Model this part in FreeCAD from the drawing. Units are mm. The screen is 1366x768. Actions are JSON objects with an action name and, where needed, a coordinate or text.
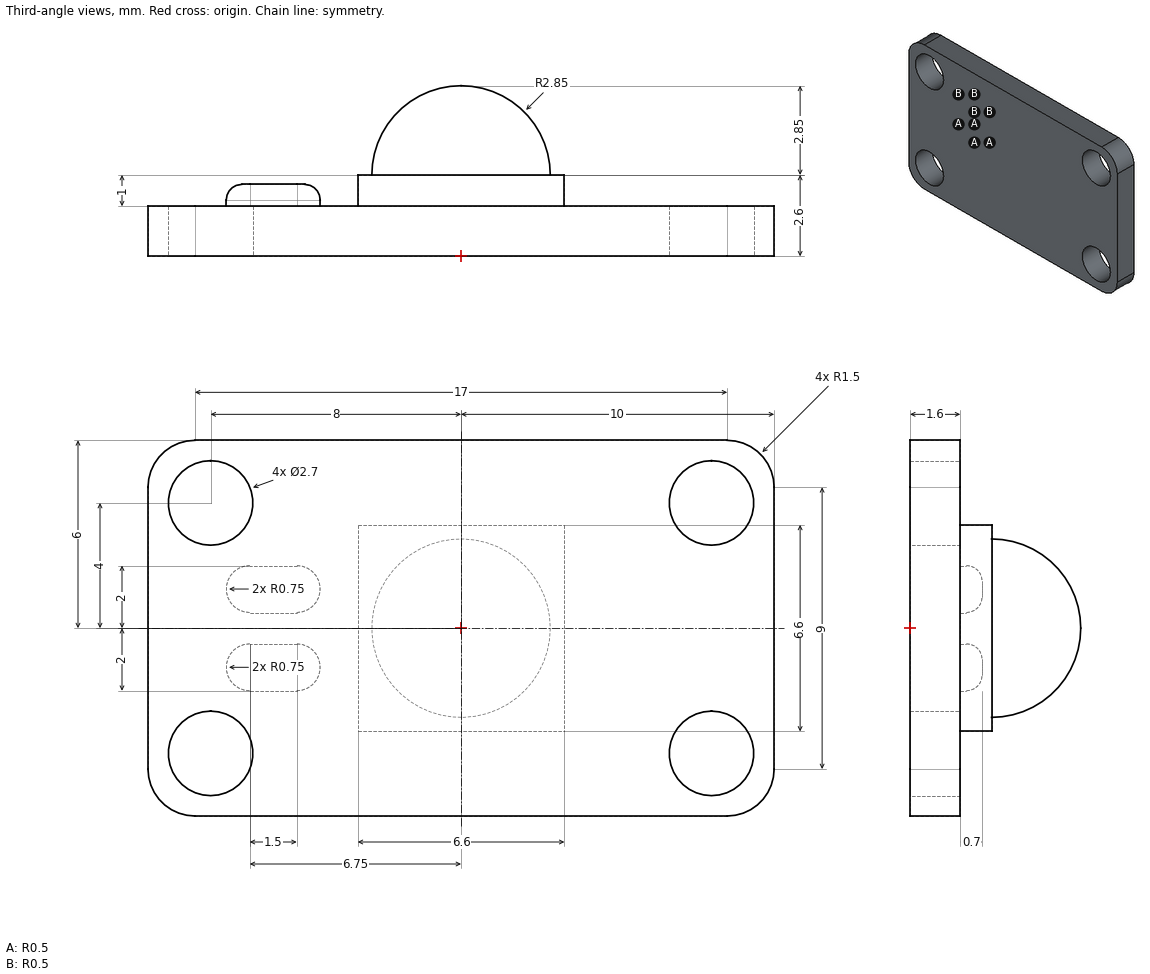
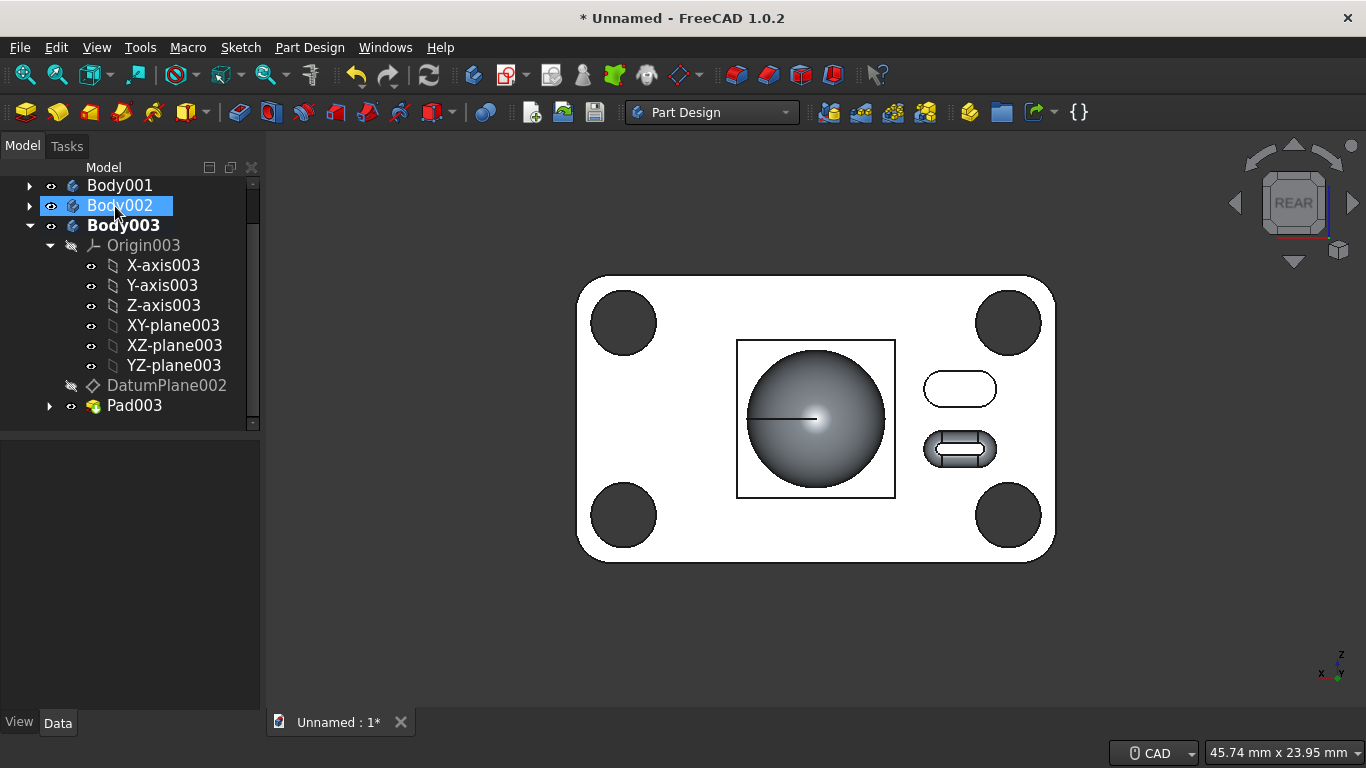
{"action": "left_click", "coordinate": [26, 76]}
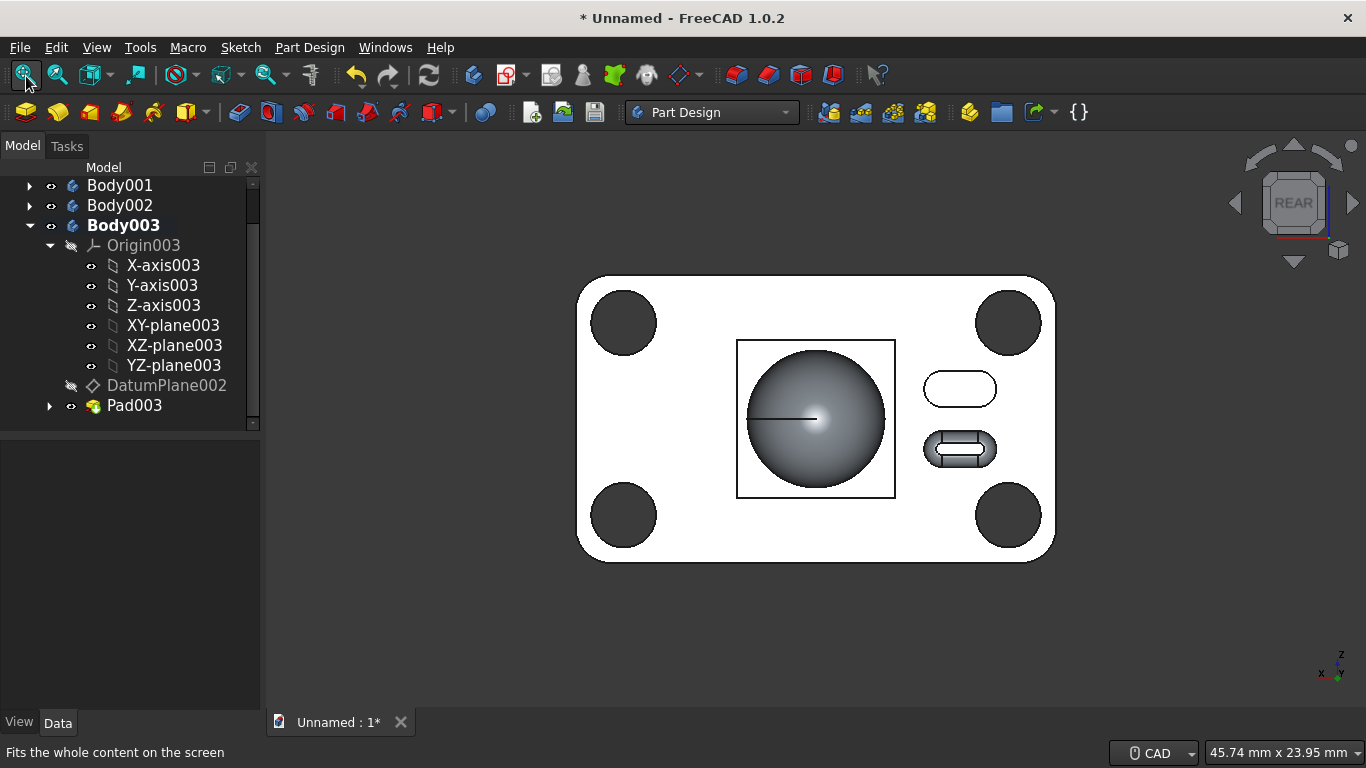
{"action": "left_click", "coordinate": [950, 388]}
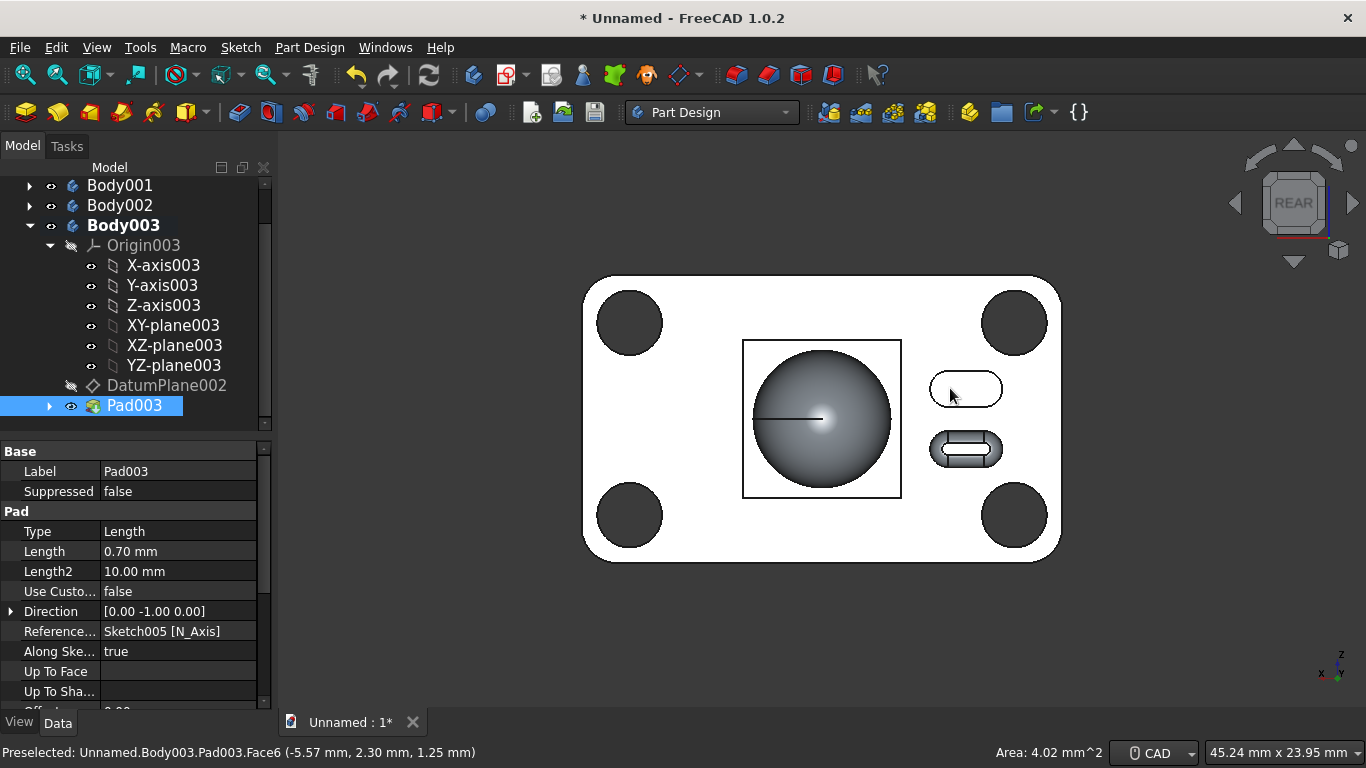
{"action": "left_click", "coordinate": [738, 76]}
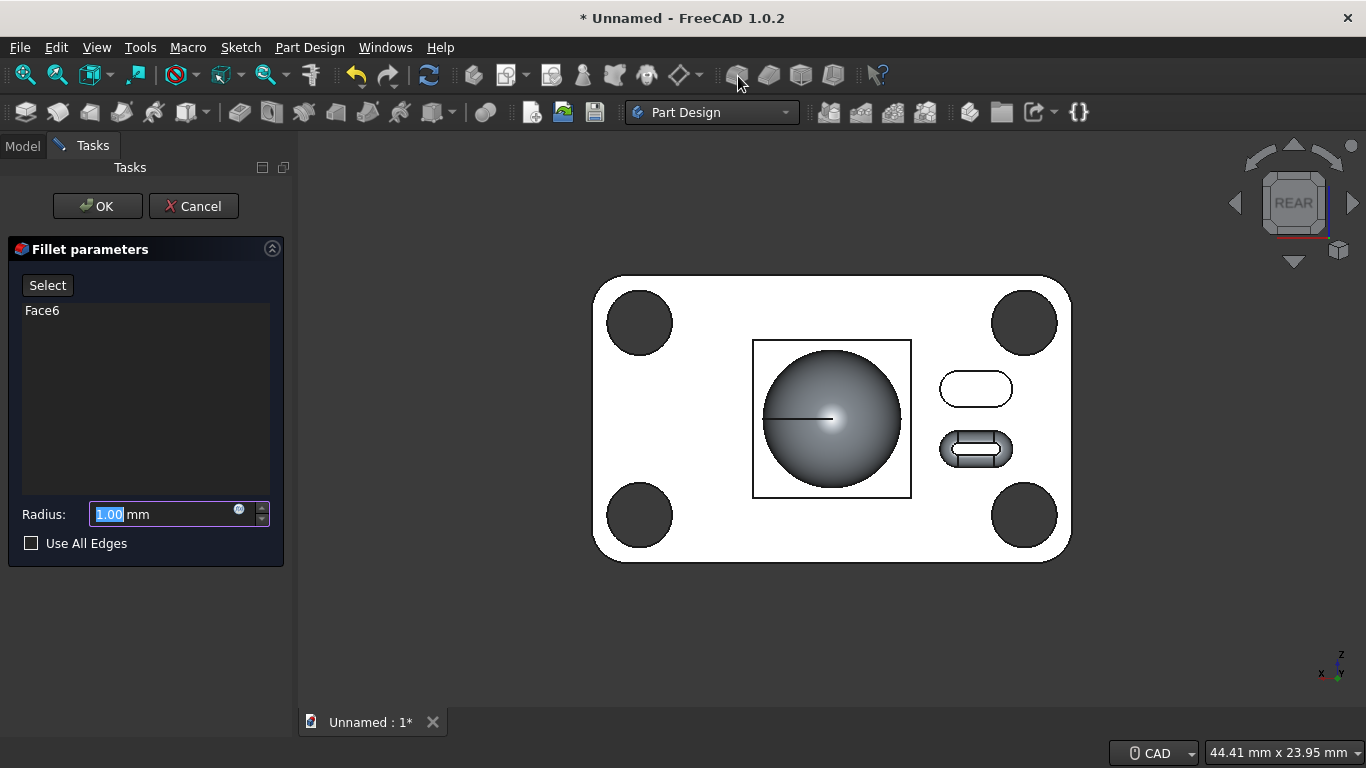
{"action": "type", "text": "0.5"}
{"action": "key", "text": "Tab"}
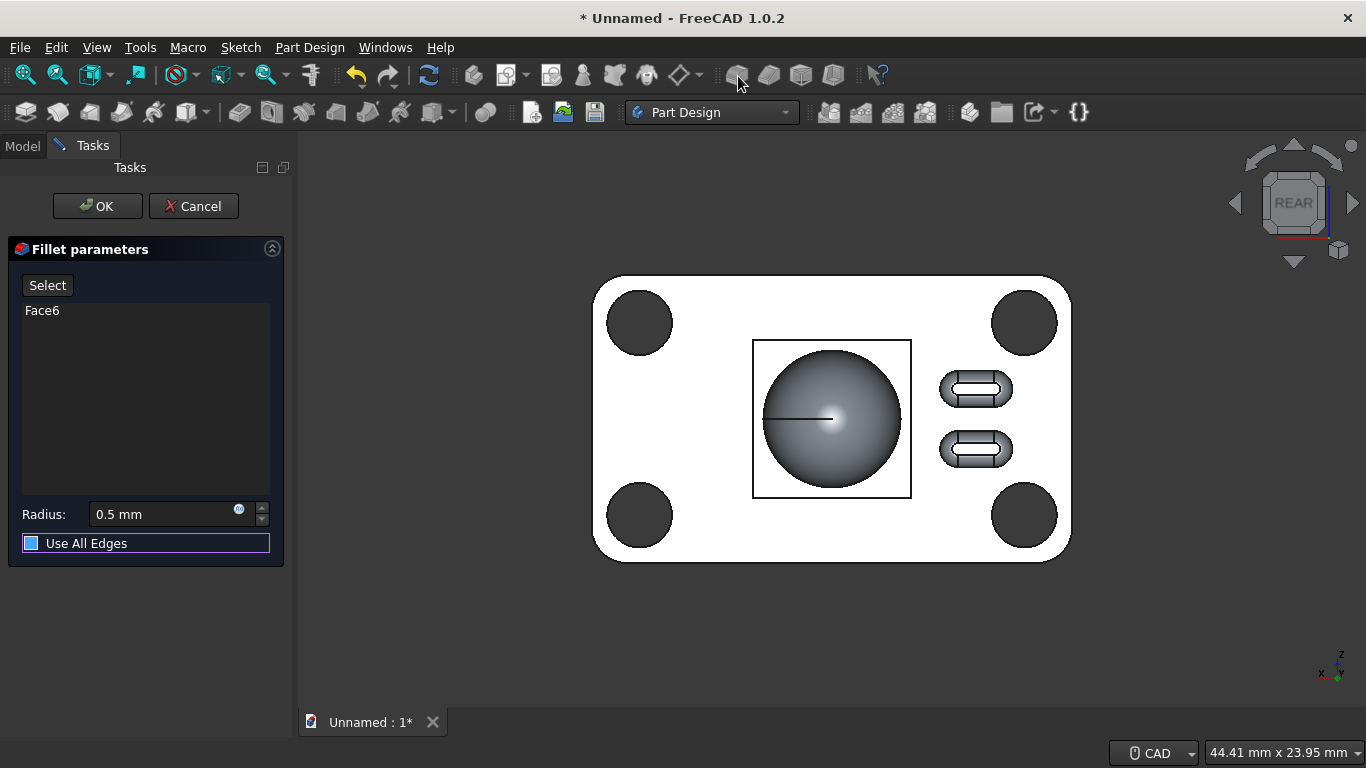
{"action": "left_click", "coordinate": [98, 206]}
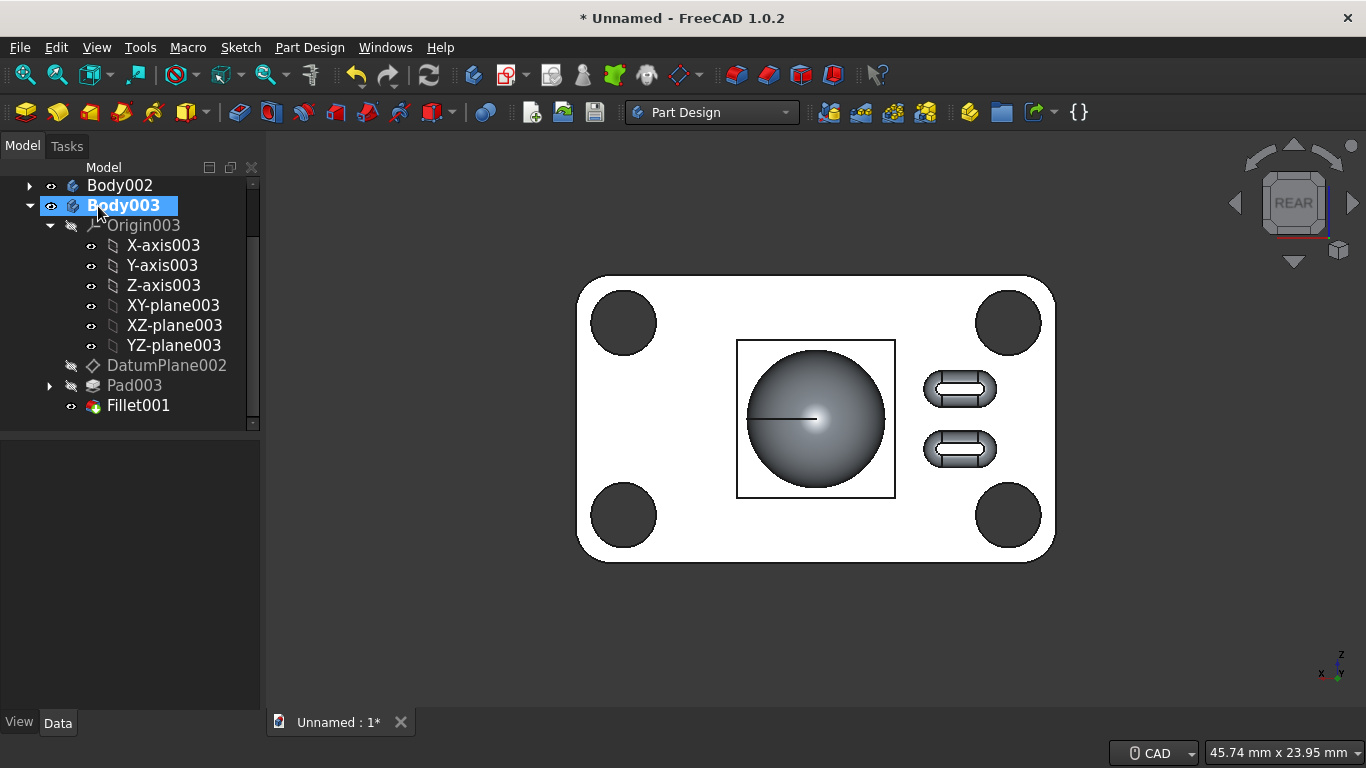
{"action": "key", "text": "0"}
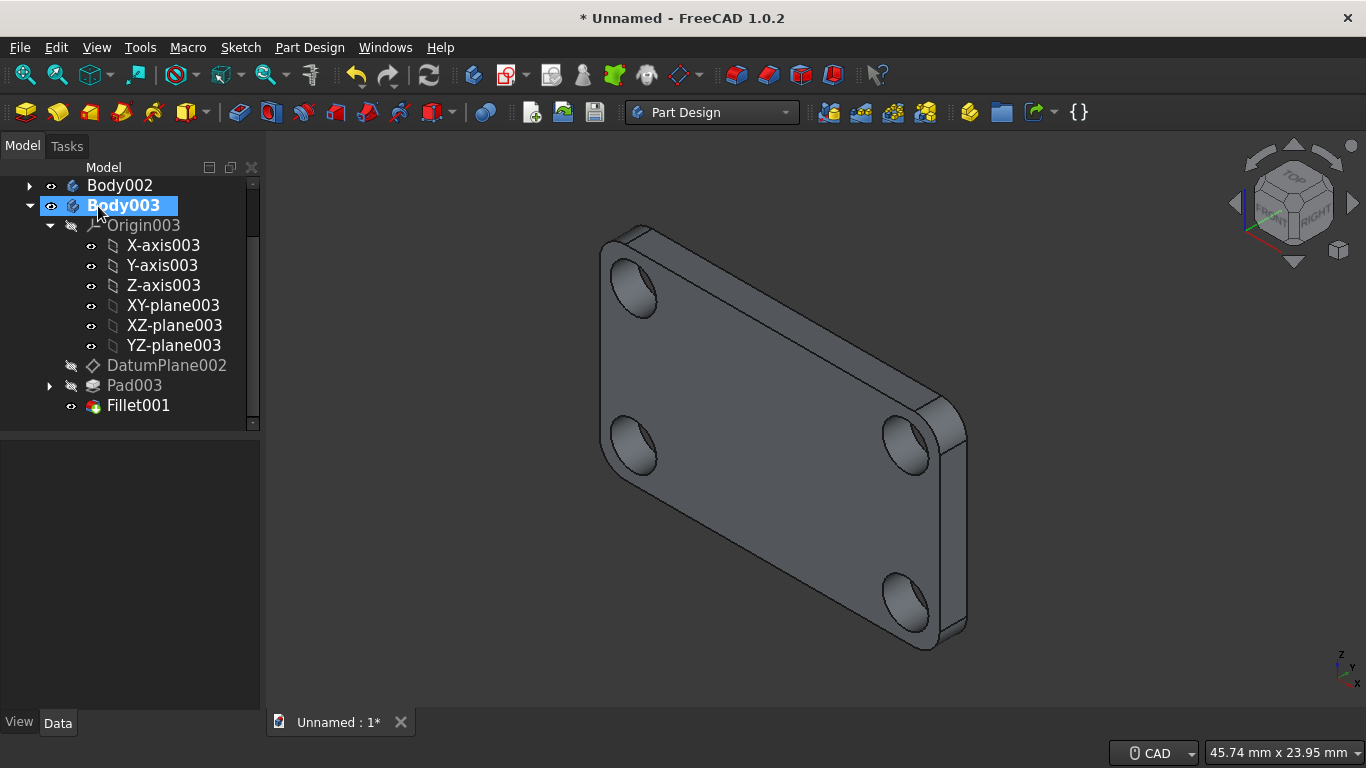
{"action": "key", "text": "v f"}